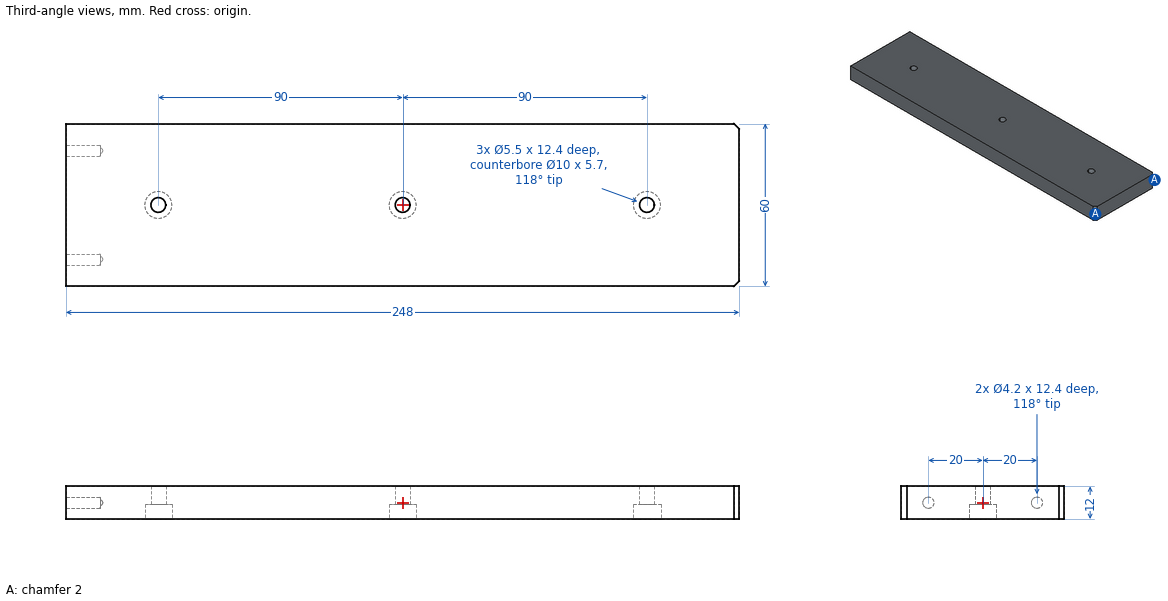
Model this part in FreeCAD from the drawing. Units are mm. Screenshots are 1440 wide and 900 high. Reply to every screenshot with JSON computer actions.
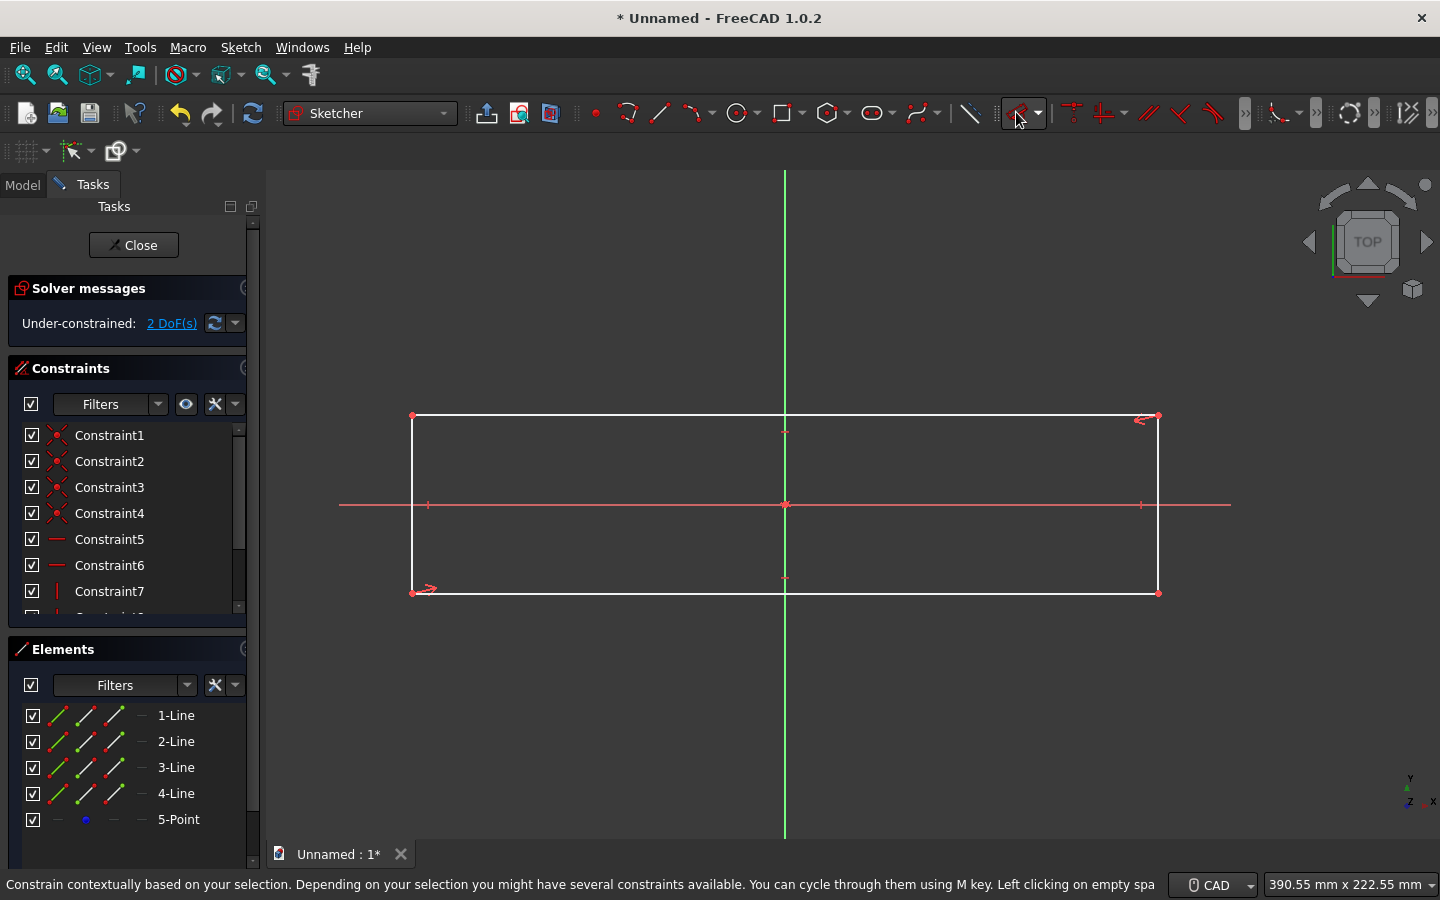
{"action": "left_click", "coordinate": [1158, 540]}
{"action": "left_click", "coordinate": [1192, 463]}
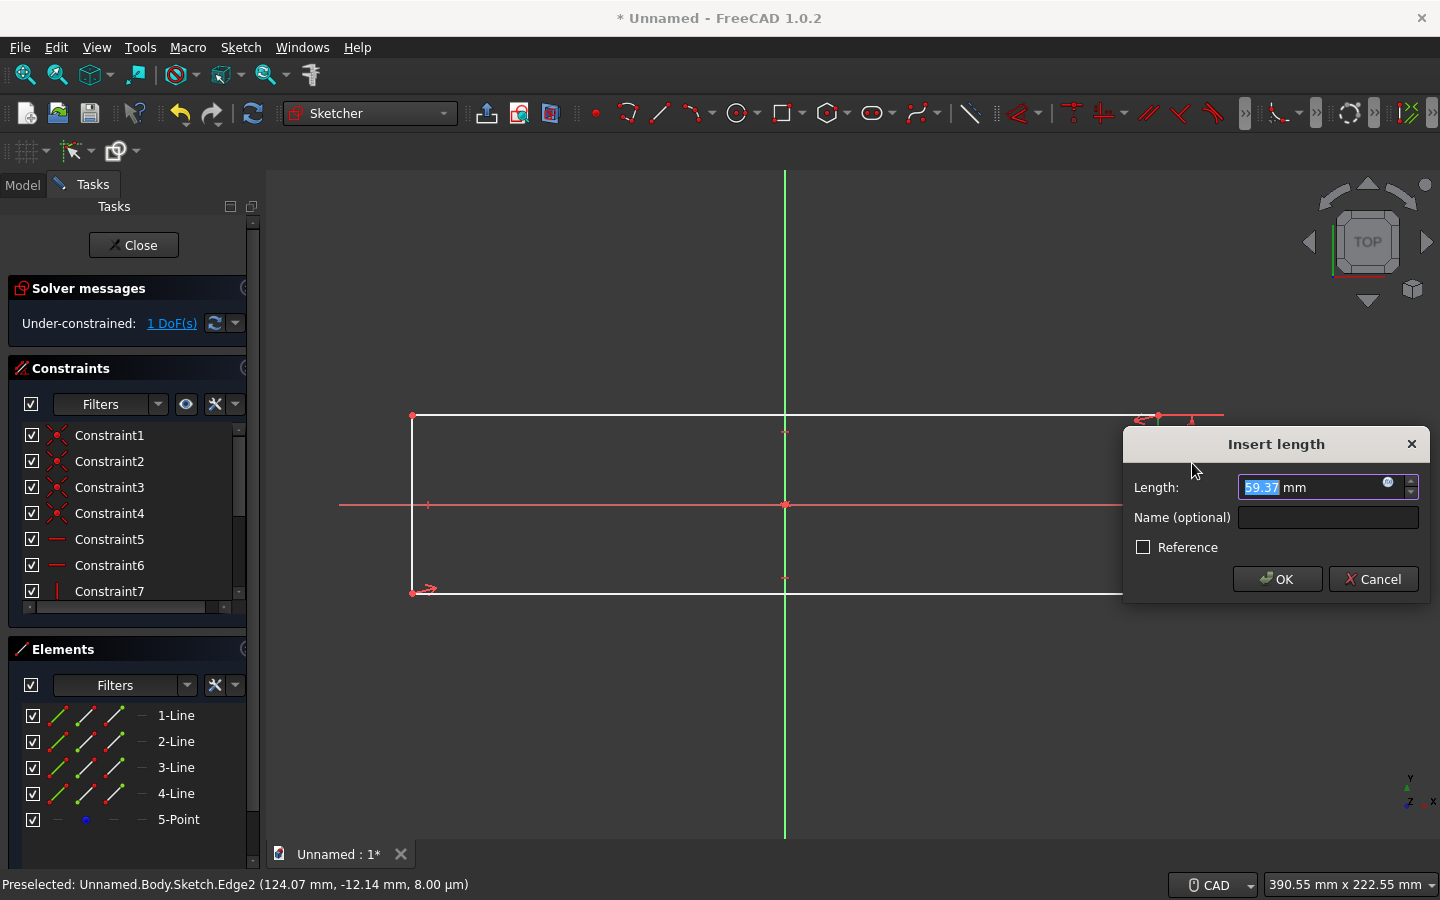
{"action": "type", "text": "60"}
{"action": "key", "text": "Return"}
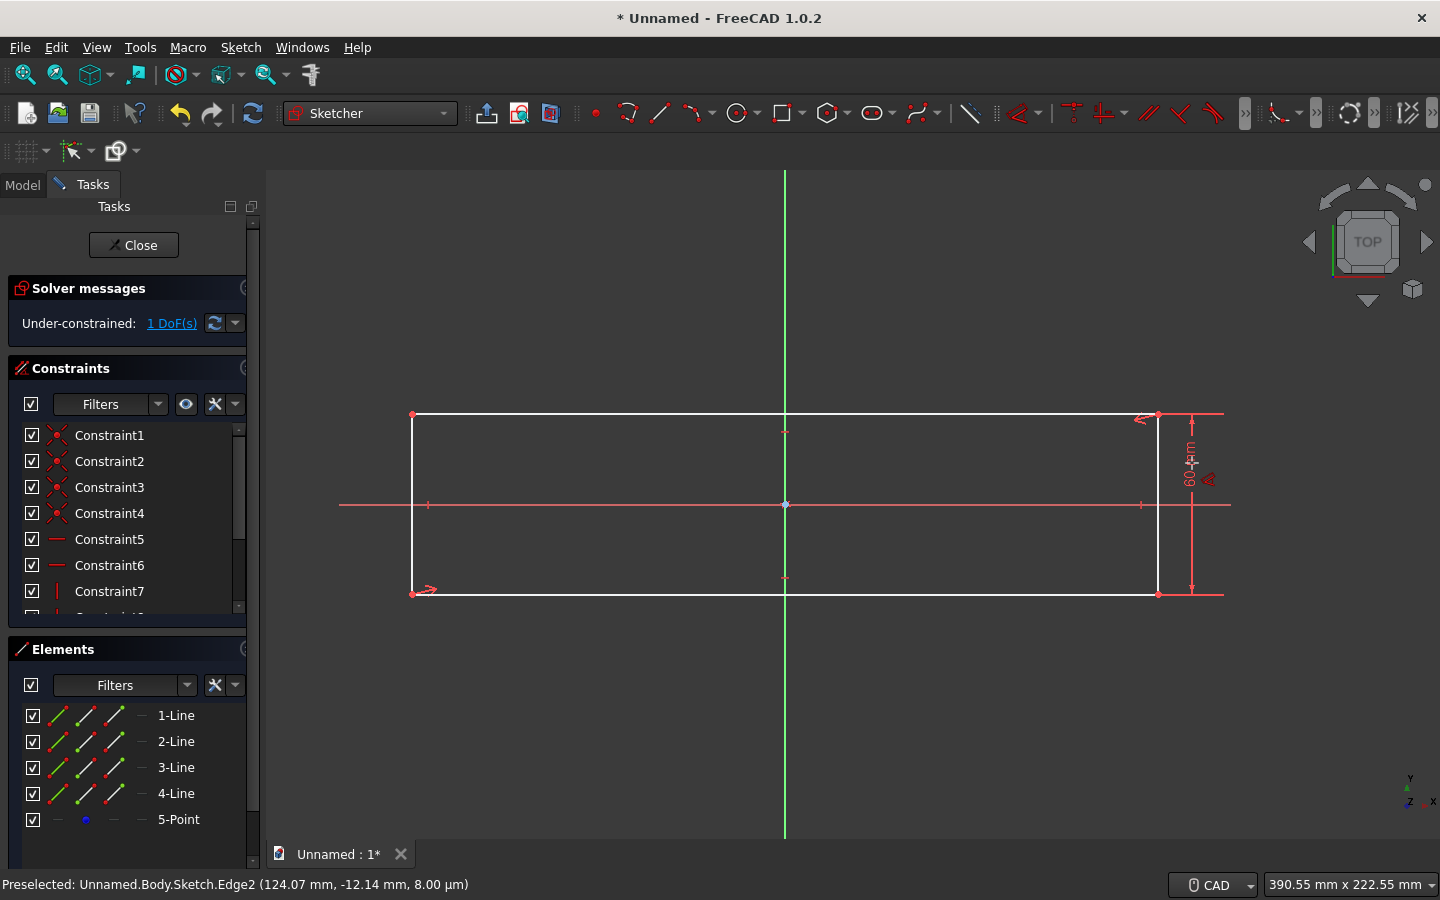
{"action": "left_click", "coordinate": [636, 595]}
{"action": "left_click", "coordinate": [614, 629]}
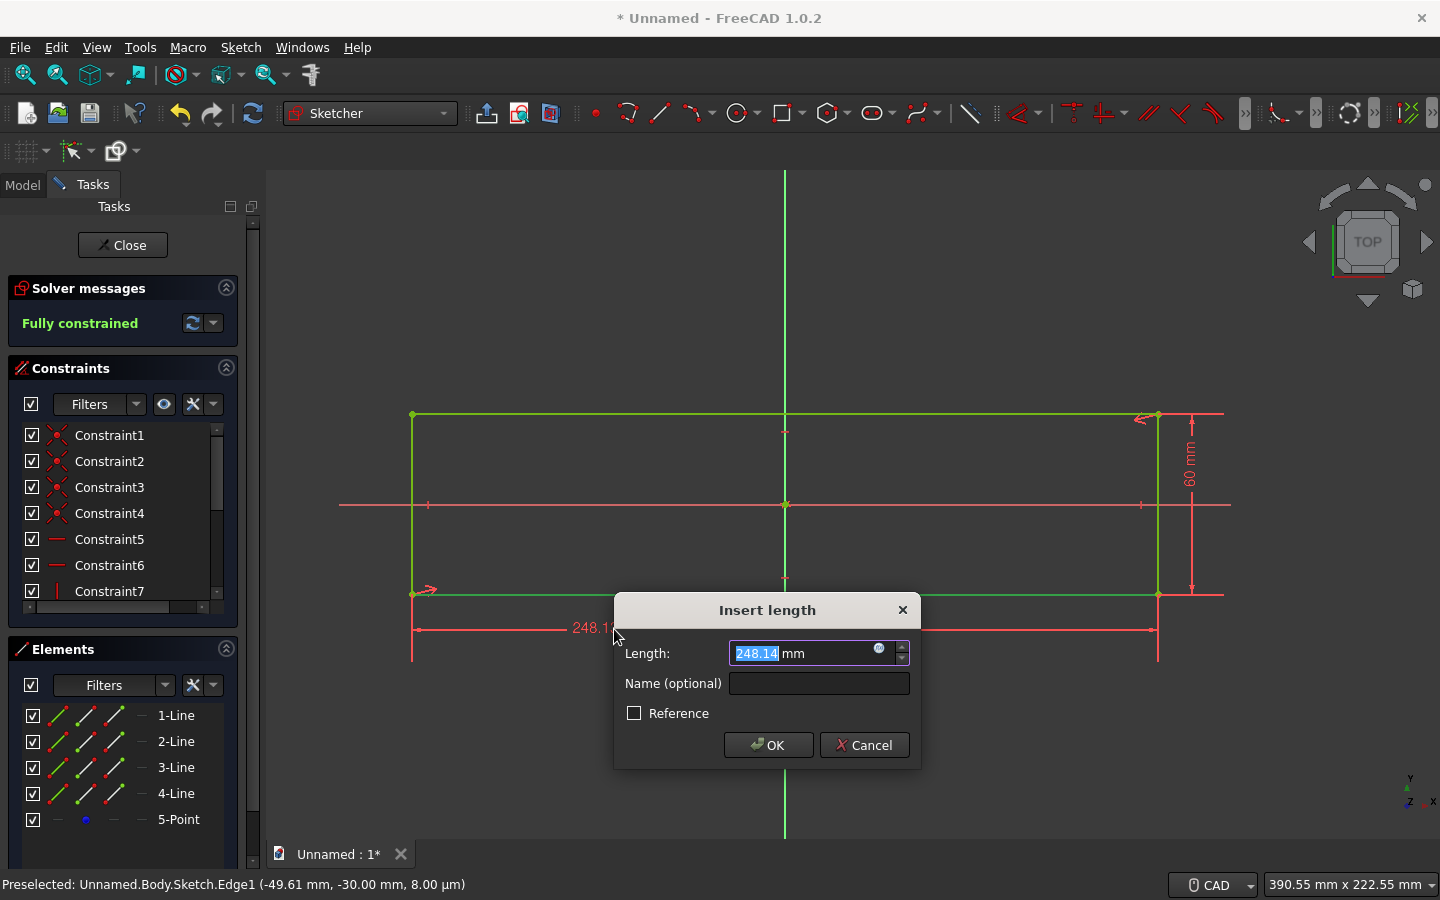
{"action": "type", "text": "248"}
{"action": "key", "text": "Return"}
{"action": "key", "text": "Escape"}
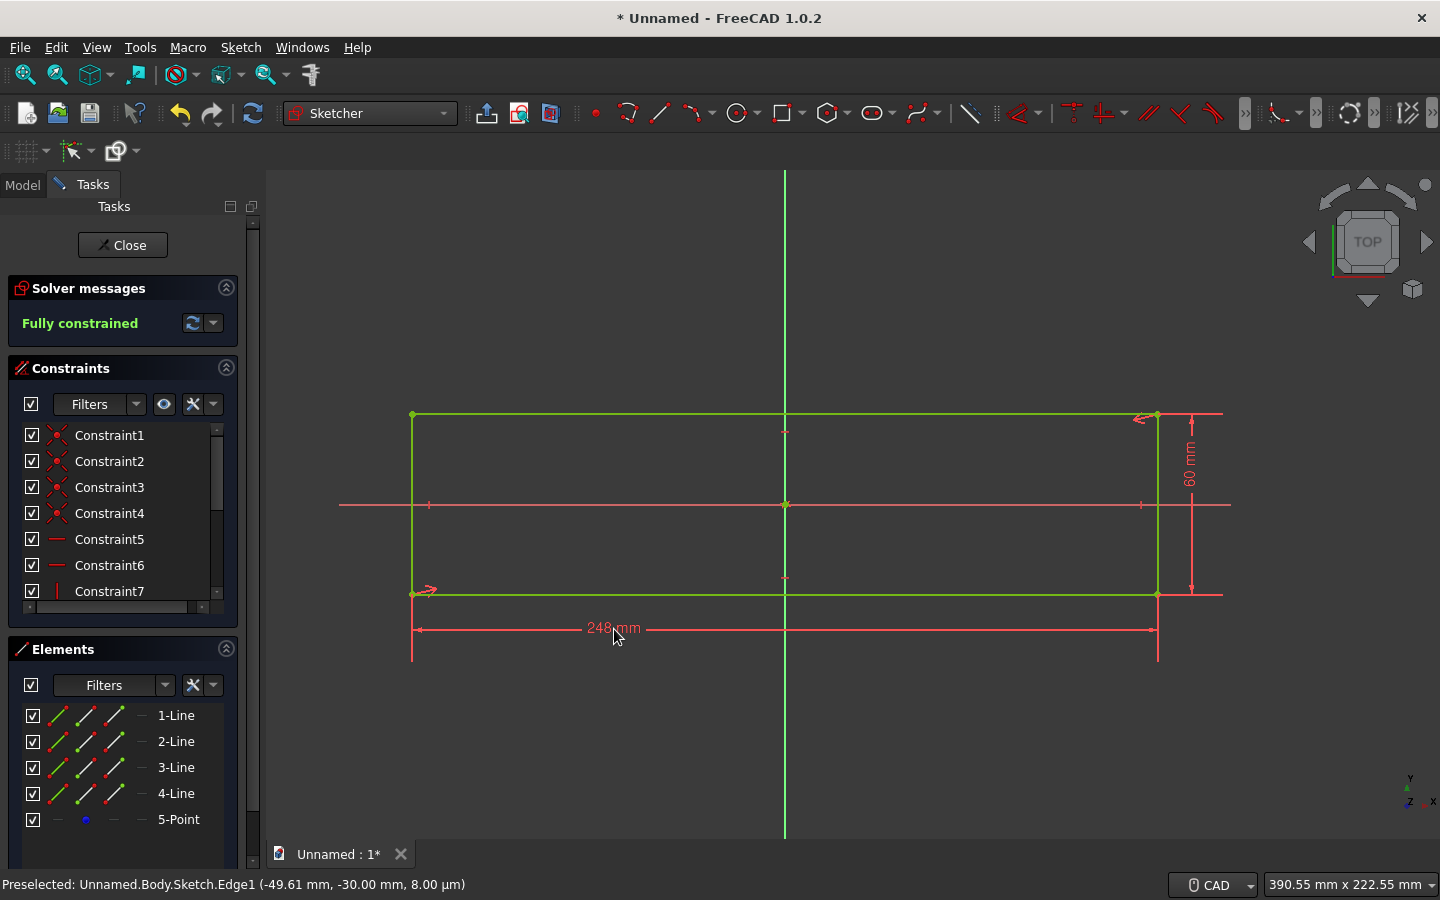
{"action": "left_click", "coordinate": [123, 245]}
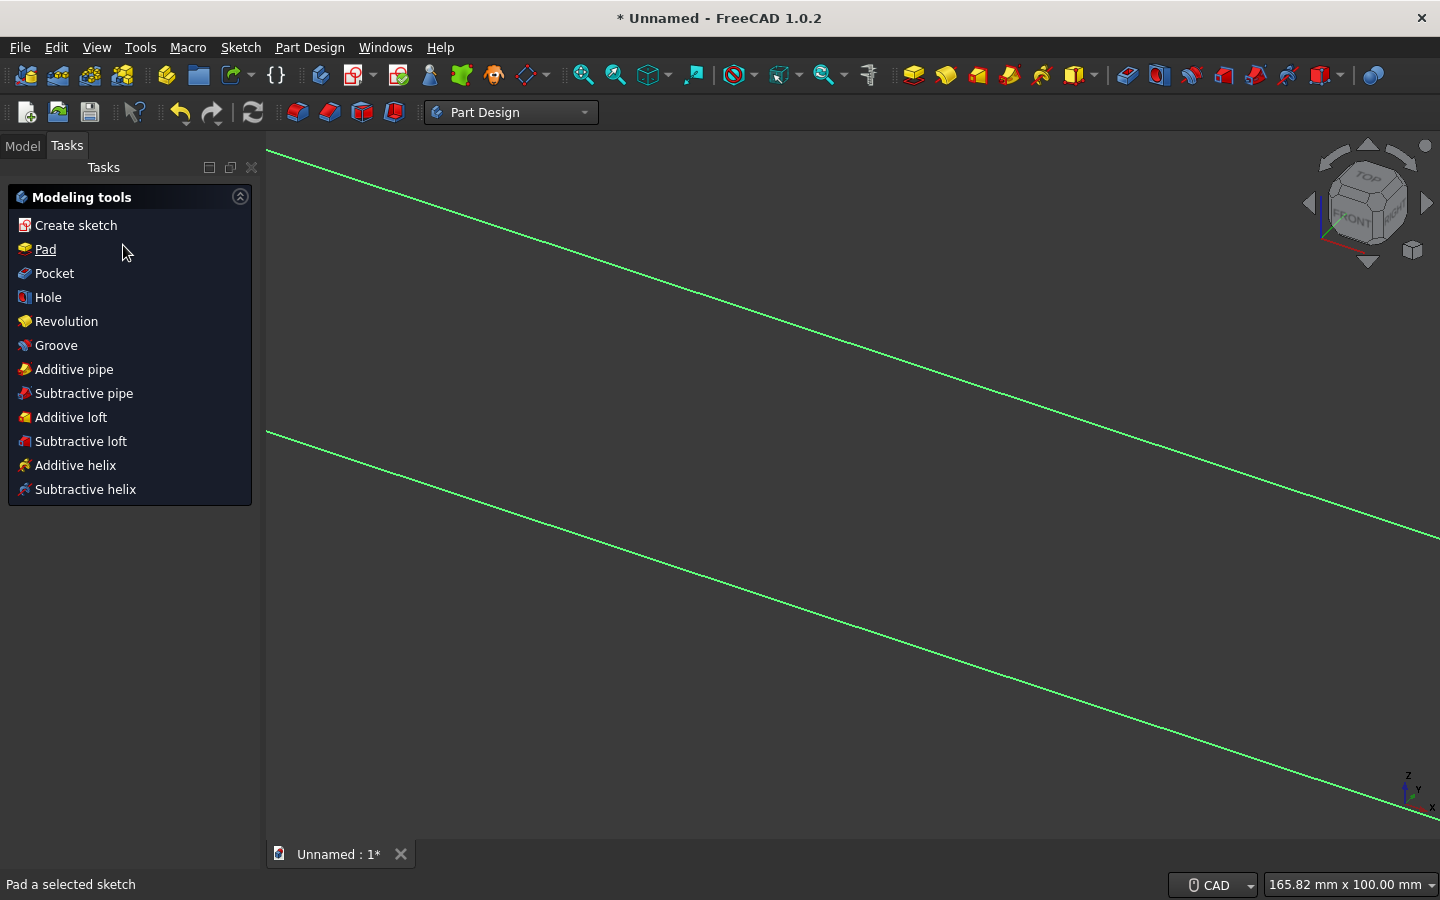
{"action": "left_click", "coordinate": [914, 76]}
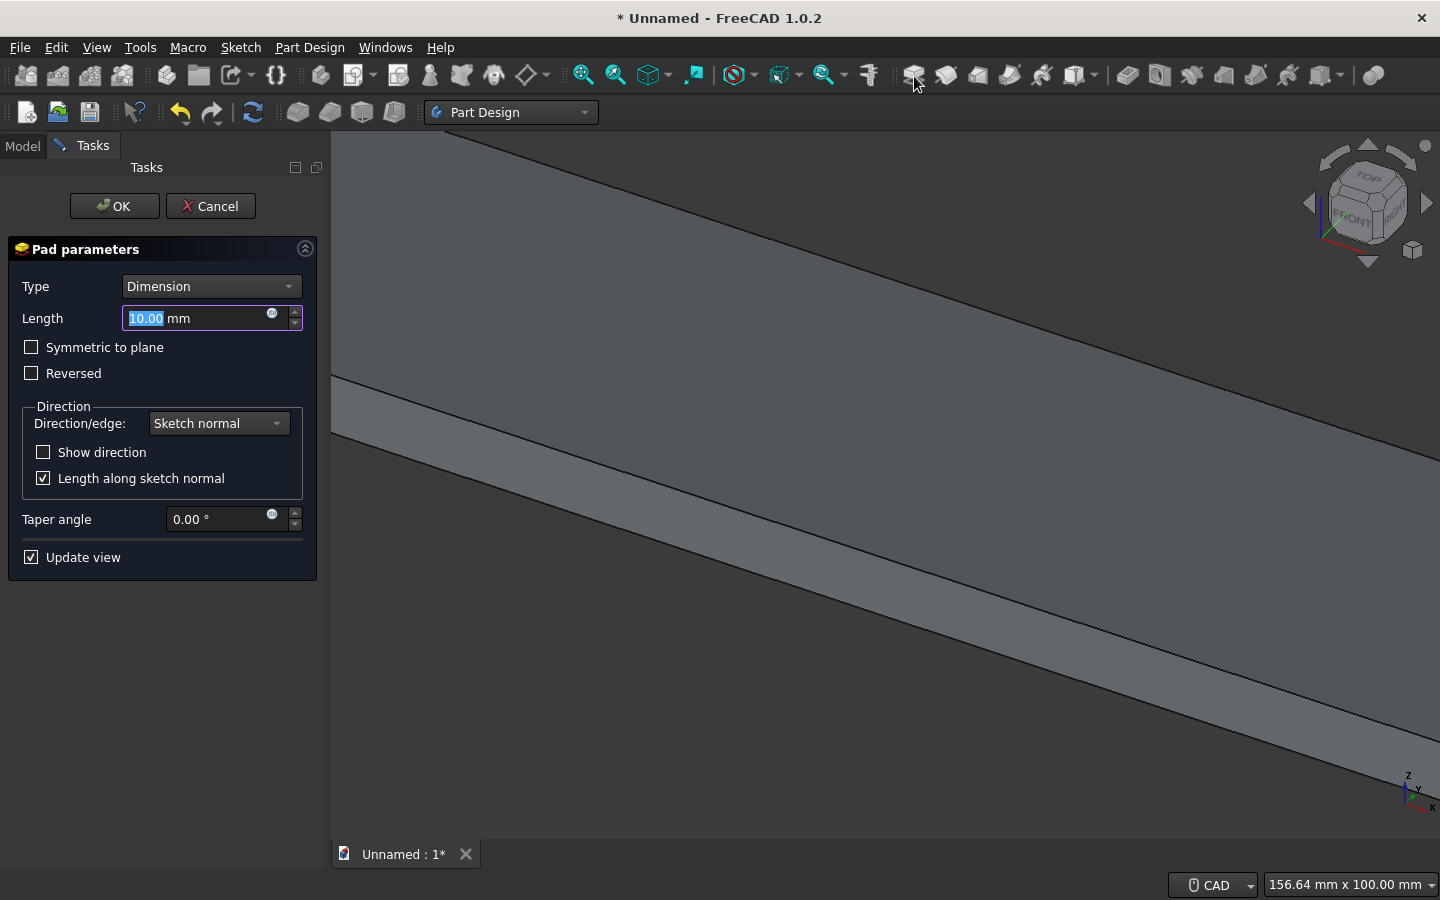
{"action": "type", "text": "12"}
{"action": "key", "text": "Tab"}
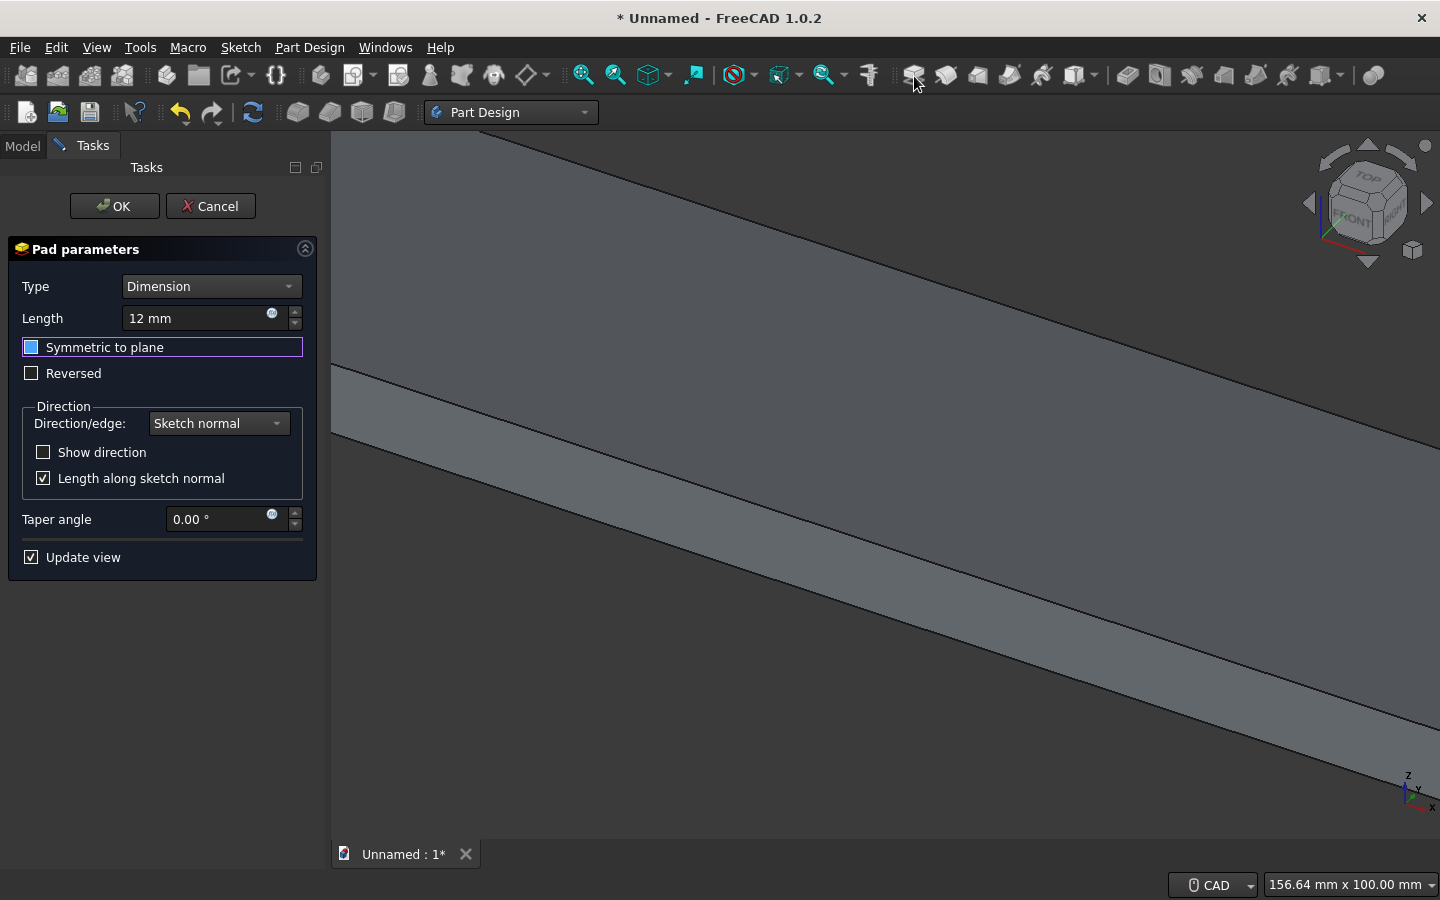
{"action": "left_click", "coordinate": [30, 347]}